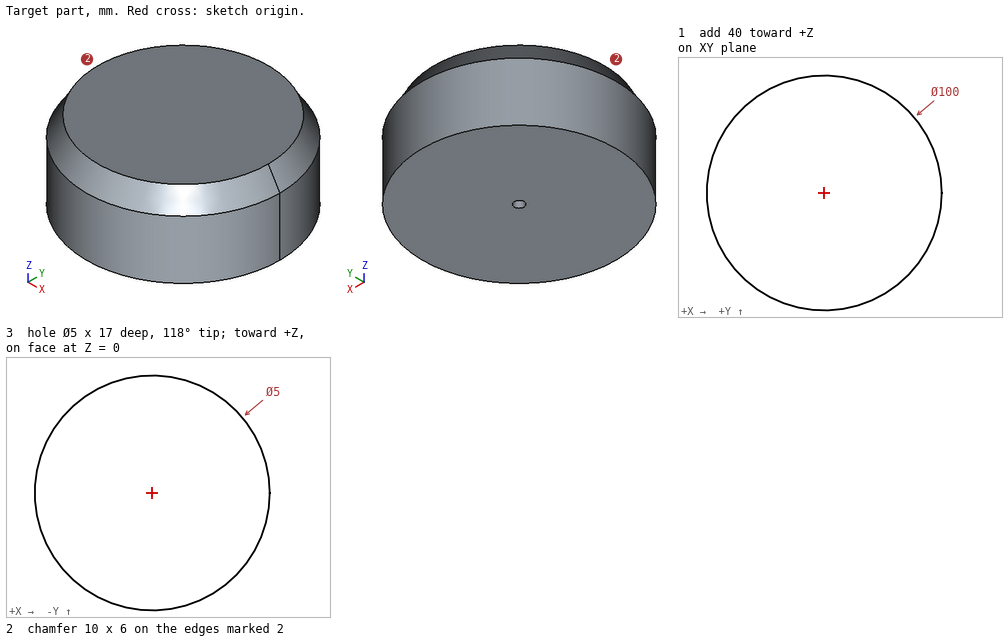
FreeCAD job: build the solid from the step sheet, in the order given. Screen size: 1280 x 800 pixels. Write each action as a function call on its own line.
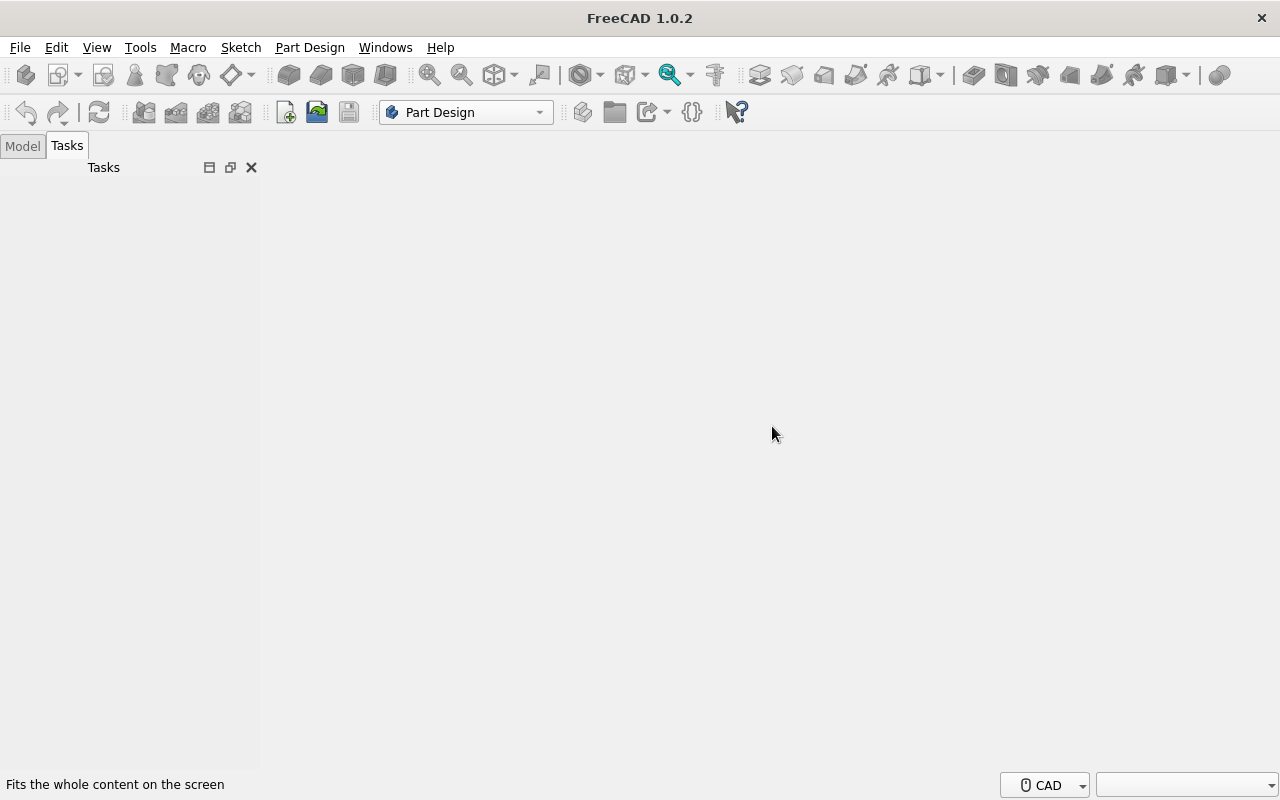
click(286, 112)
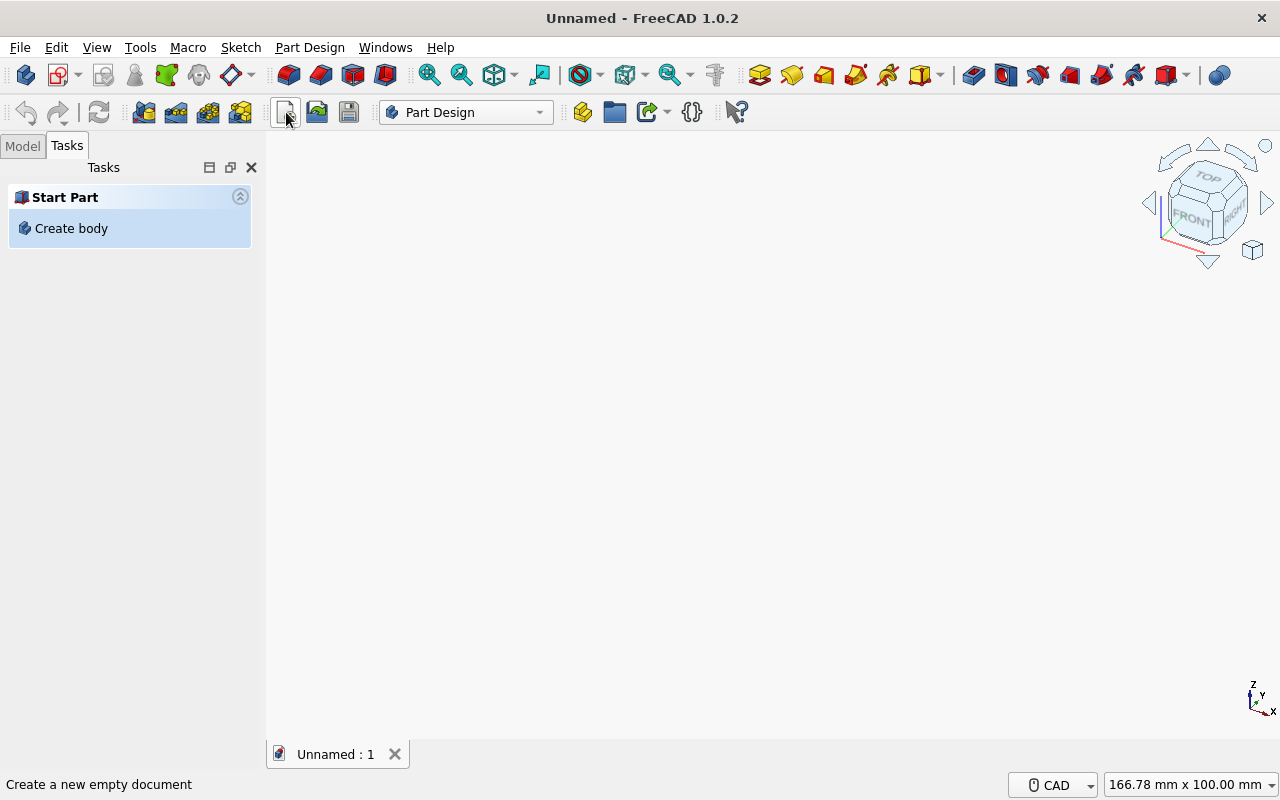
click(58, 76)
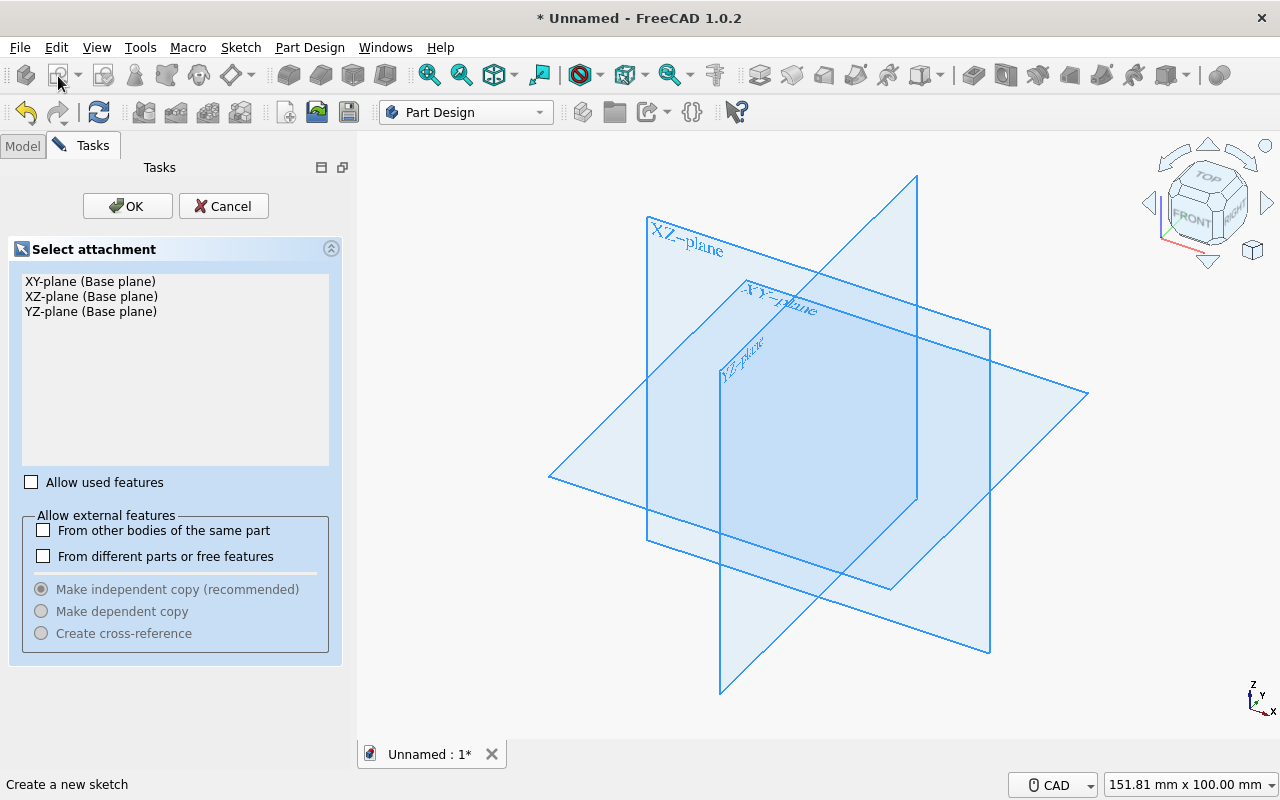
click(82, 282)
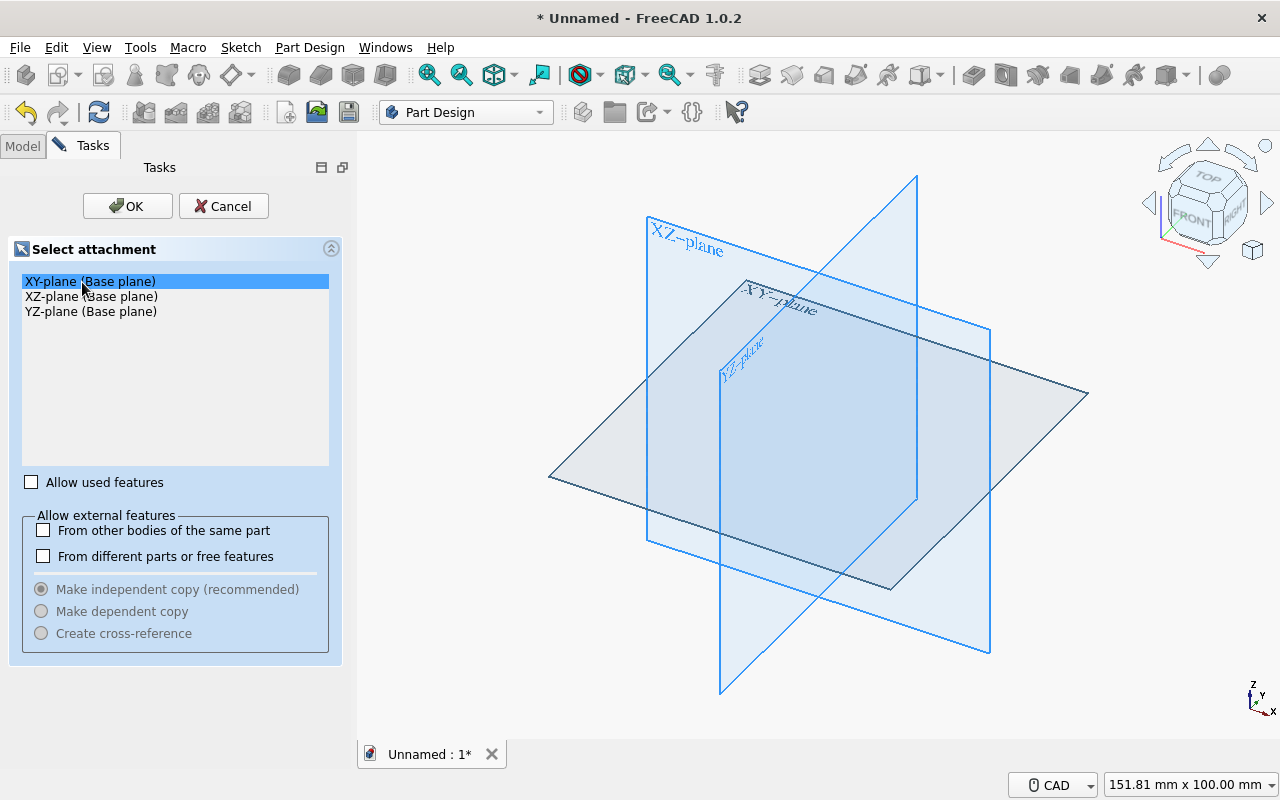
click(128, 206)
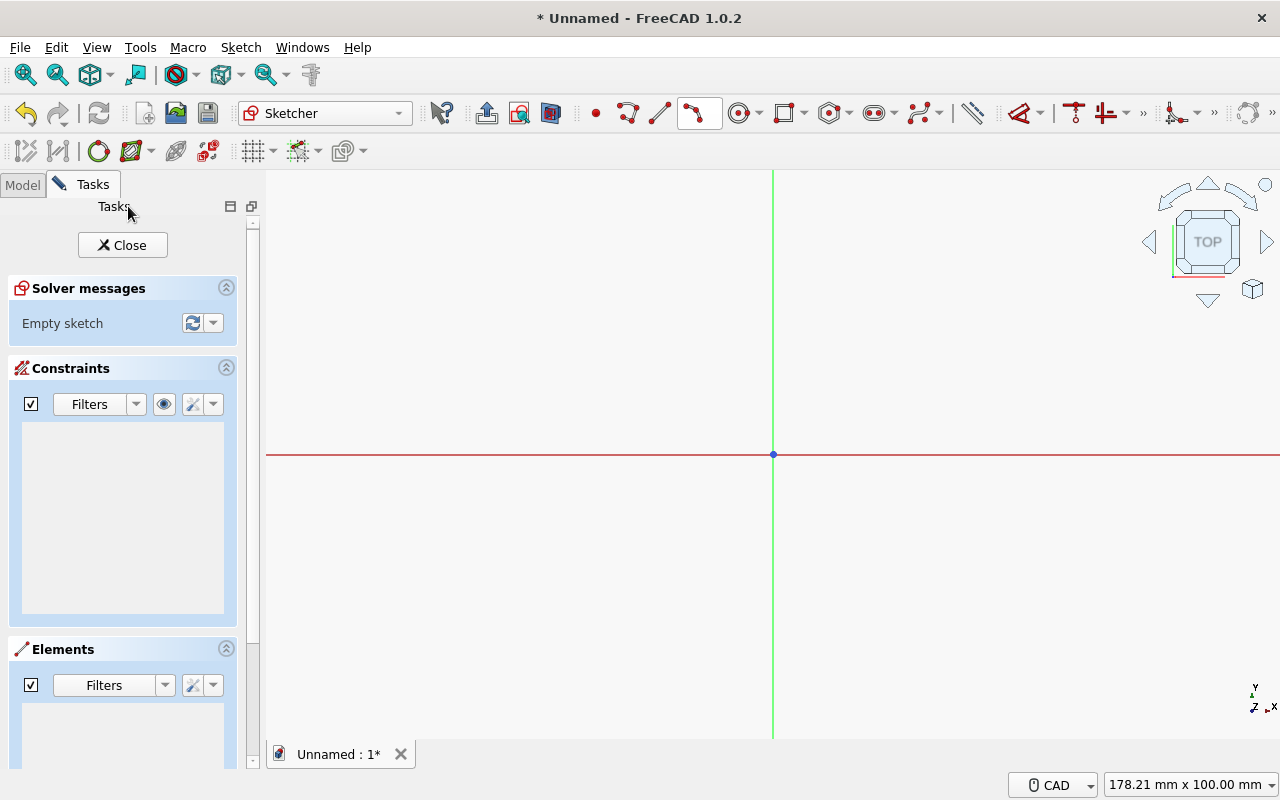
scroll(565, 455, down, 2)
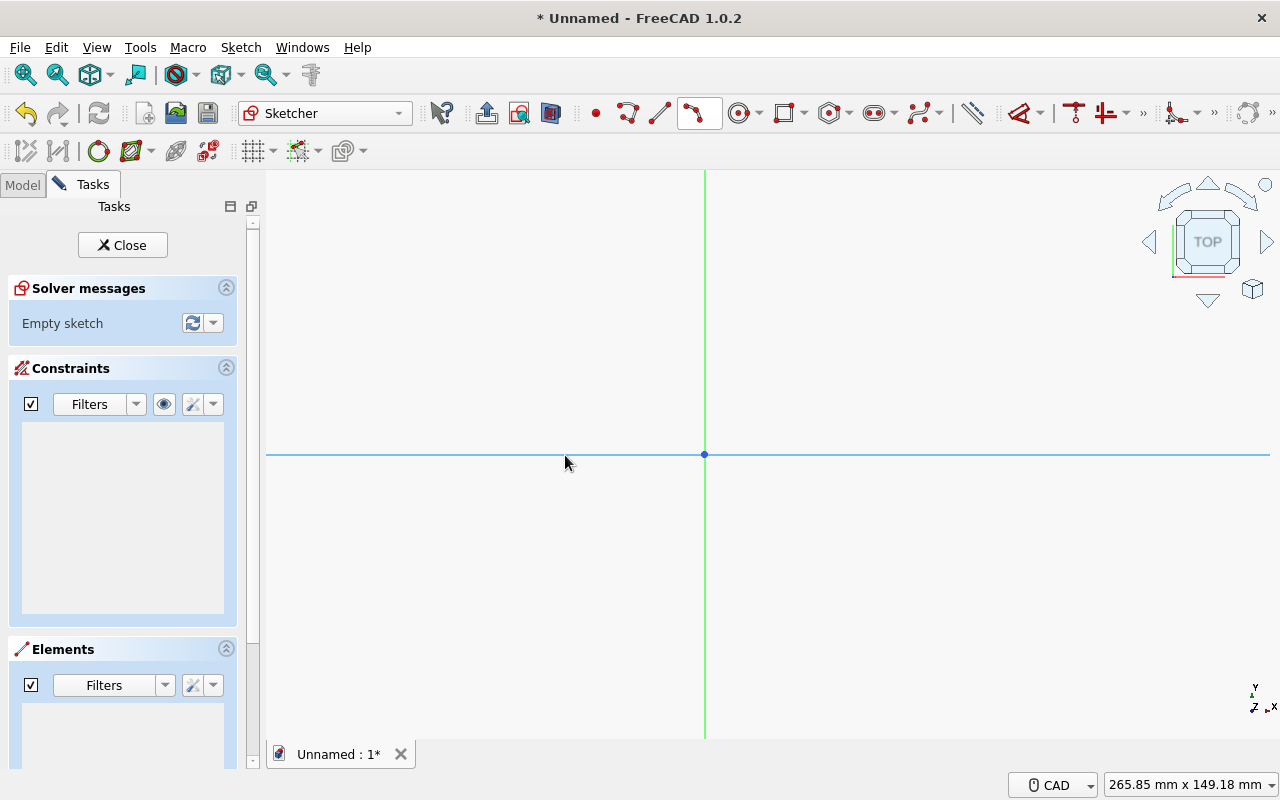
click(740, 114)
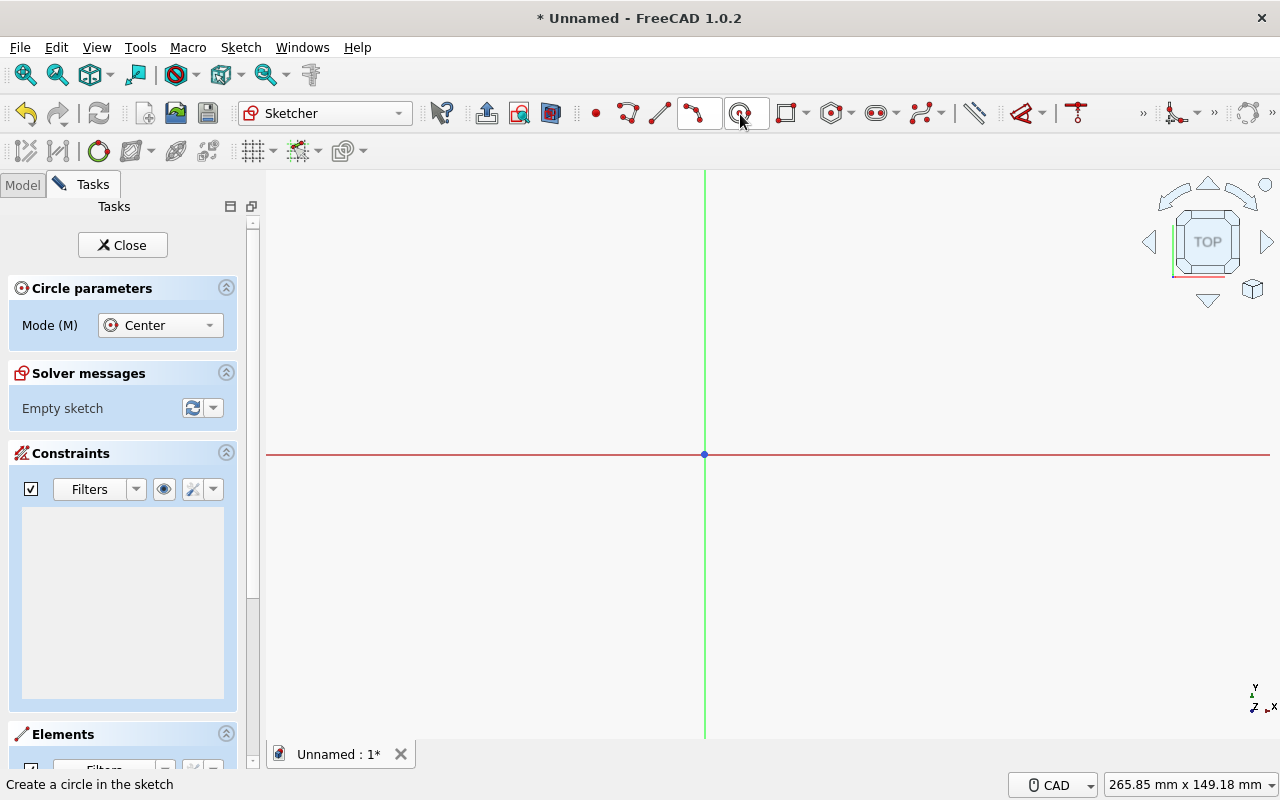
click(705, 455)
click(839, 320)
key(Escape)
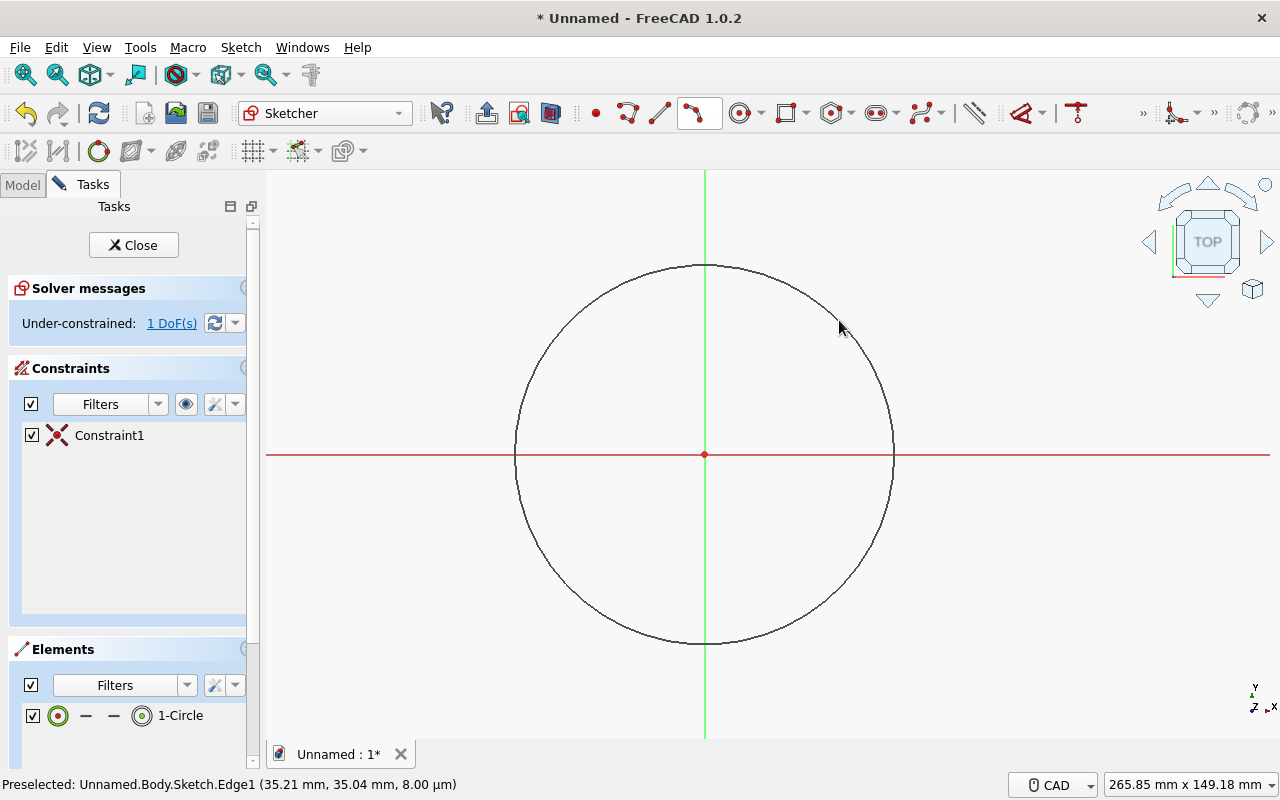
click(838, 320)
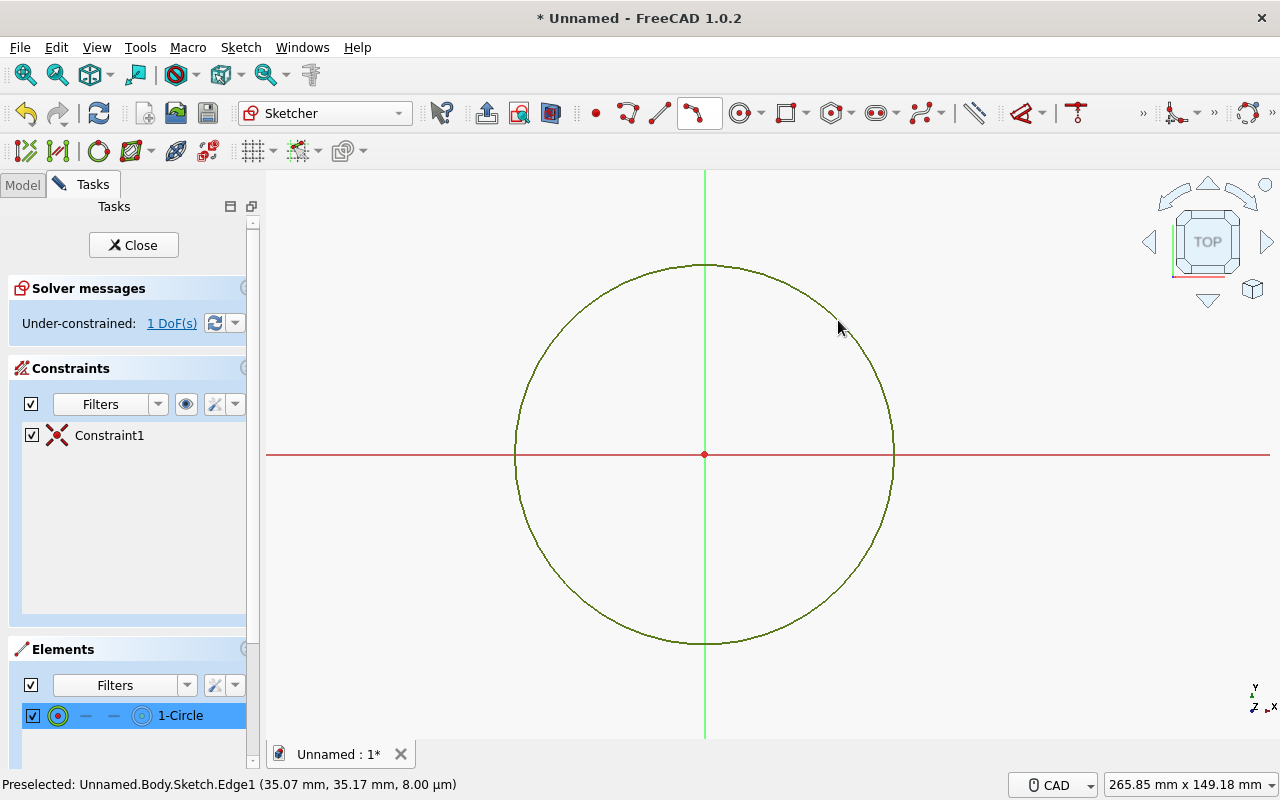
click(1044, 114)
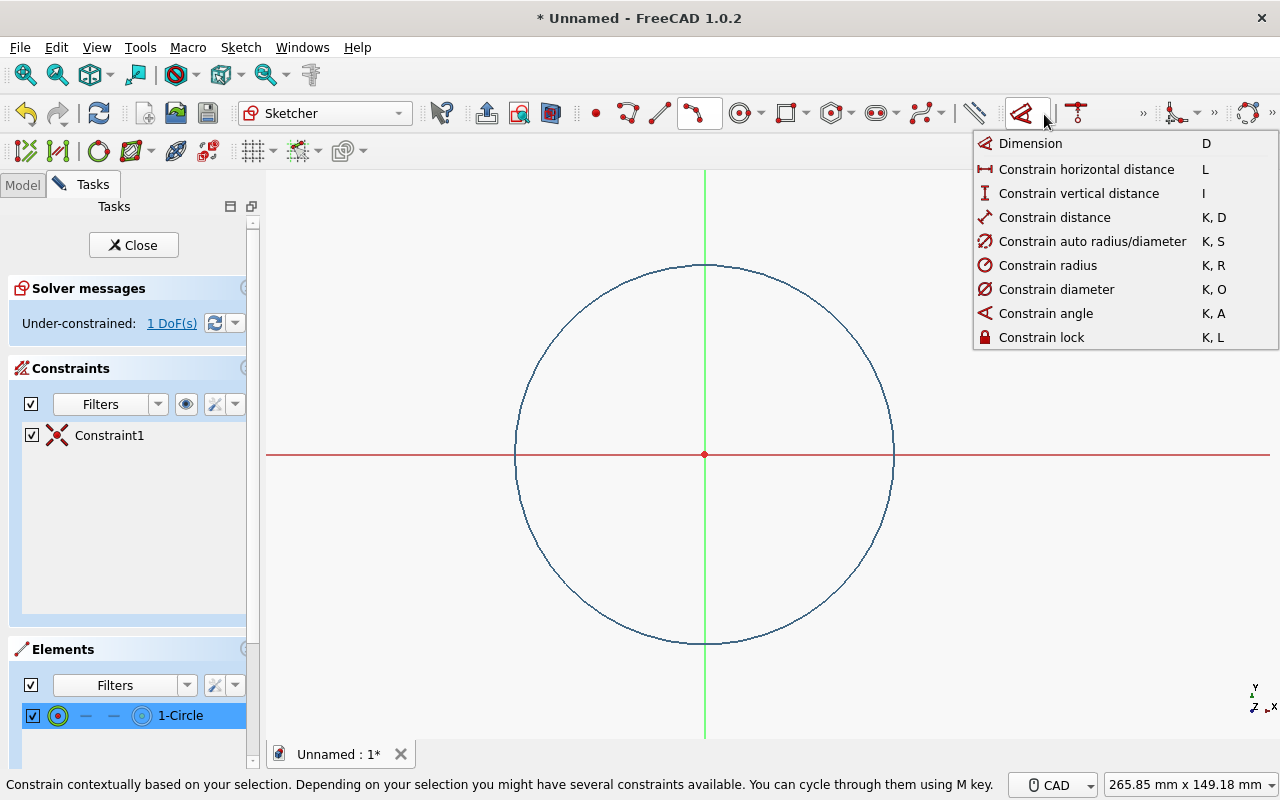
click(1126, 289)